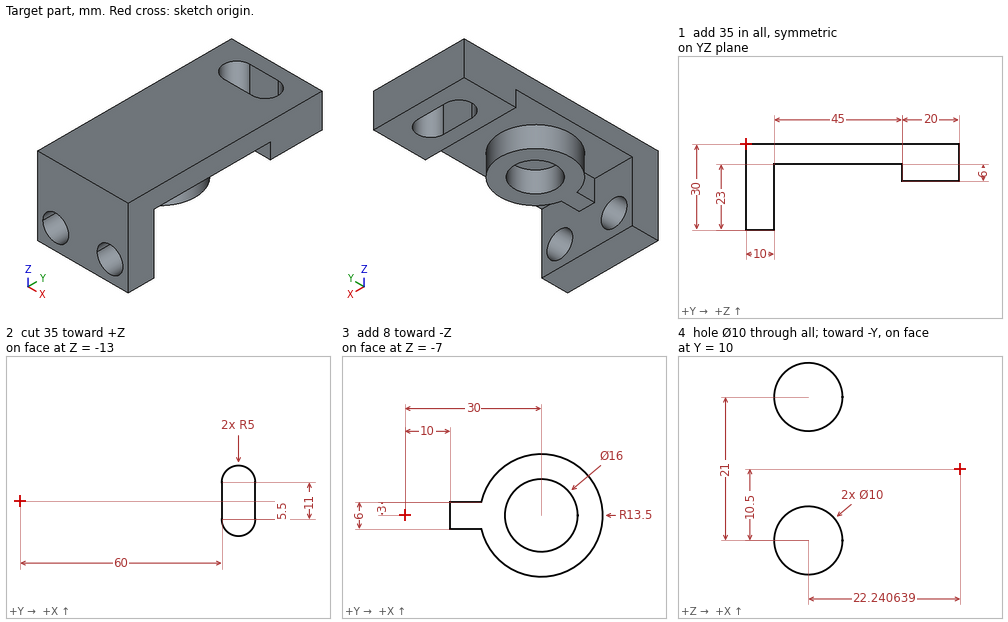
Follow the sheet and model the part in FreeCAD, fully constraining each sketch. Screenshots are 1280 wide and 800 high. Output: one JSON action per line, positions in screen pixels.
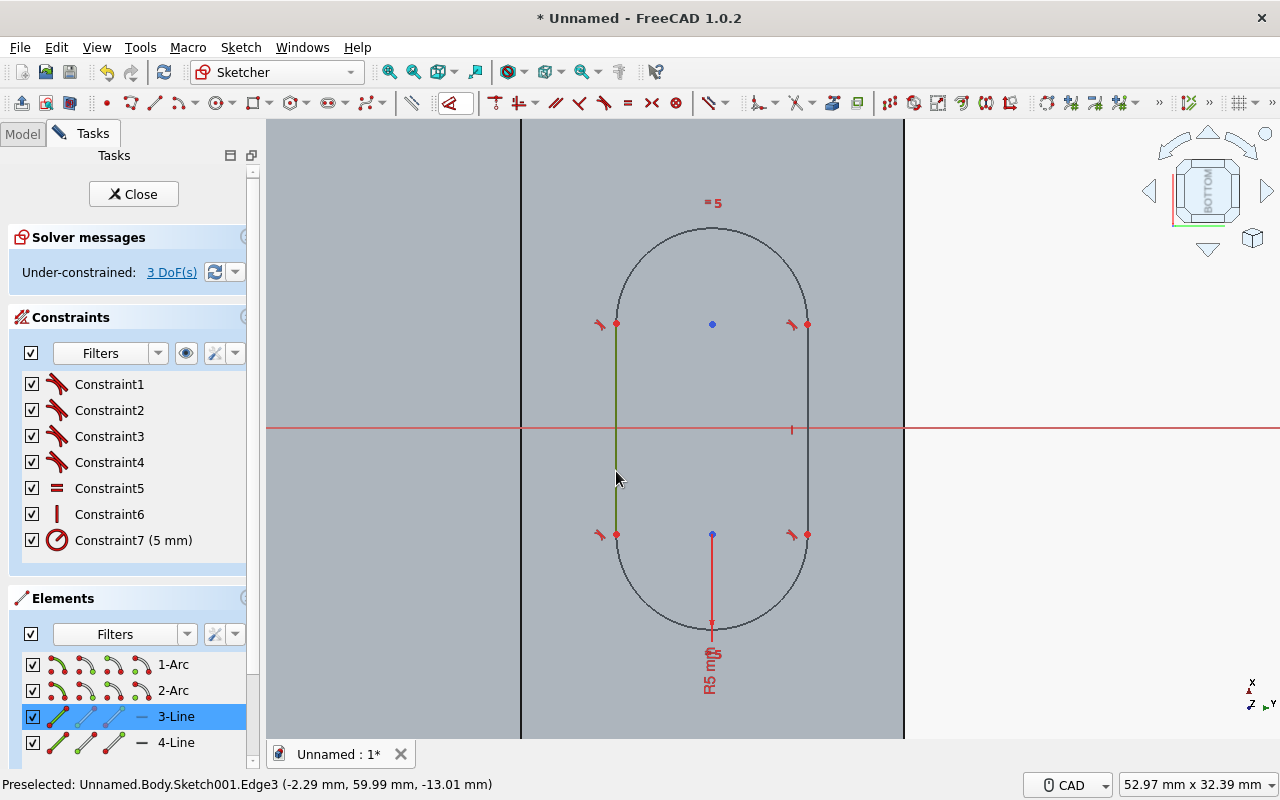
{"action": "left_click", "coordinate": [468, 104]}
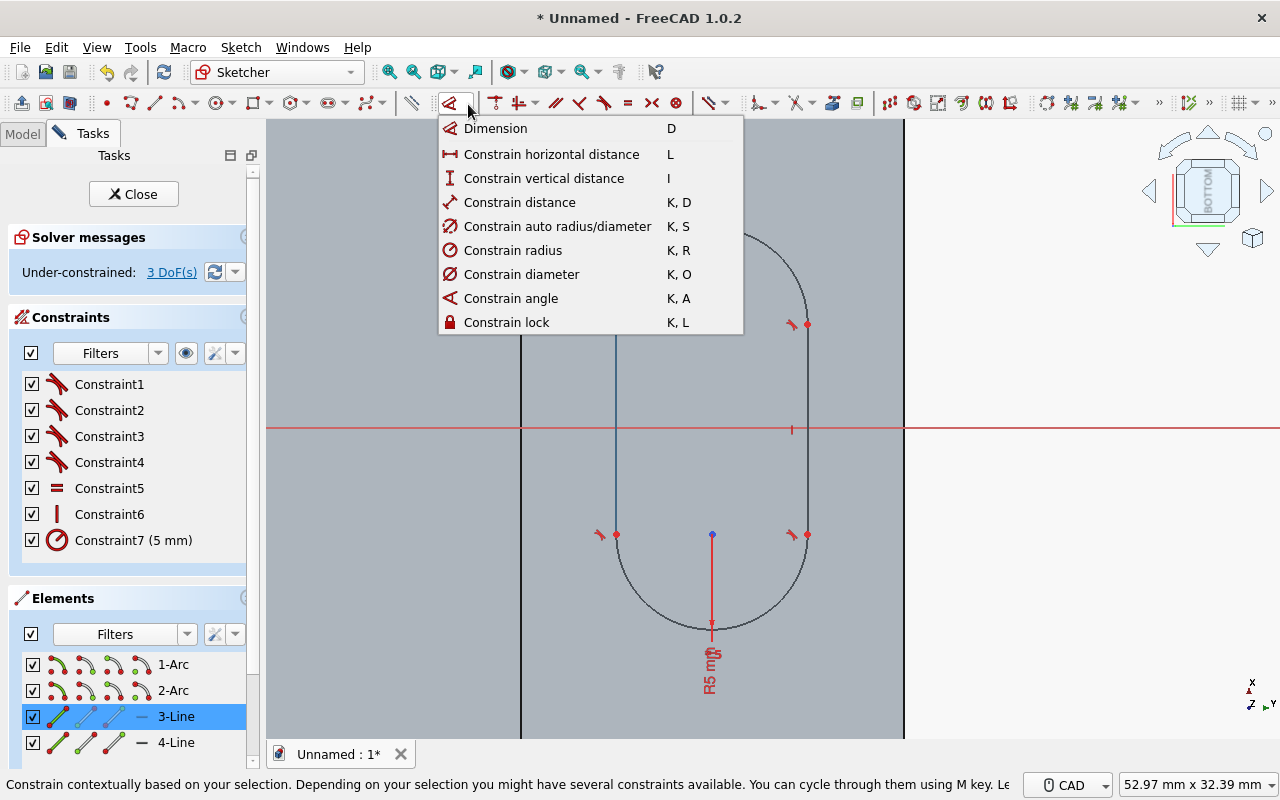
{"action": "left_click", "coordinate": [591, 178]}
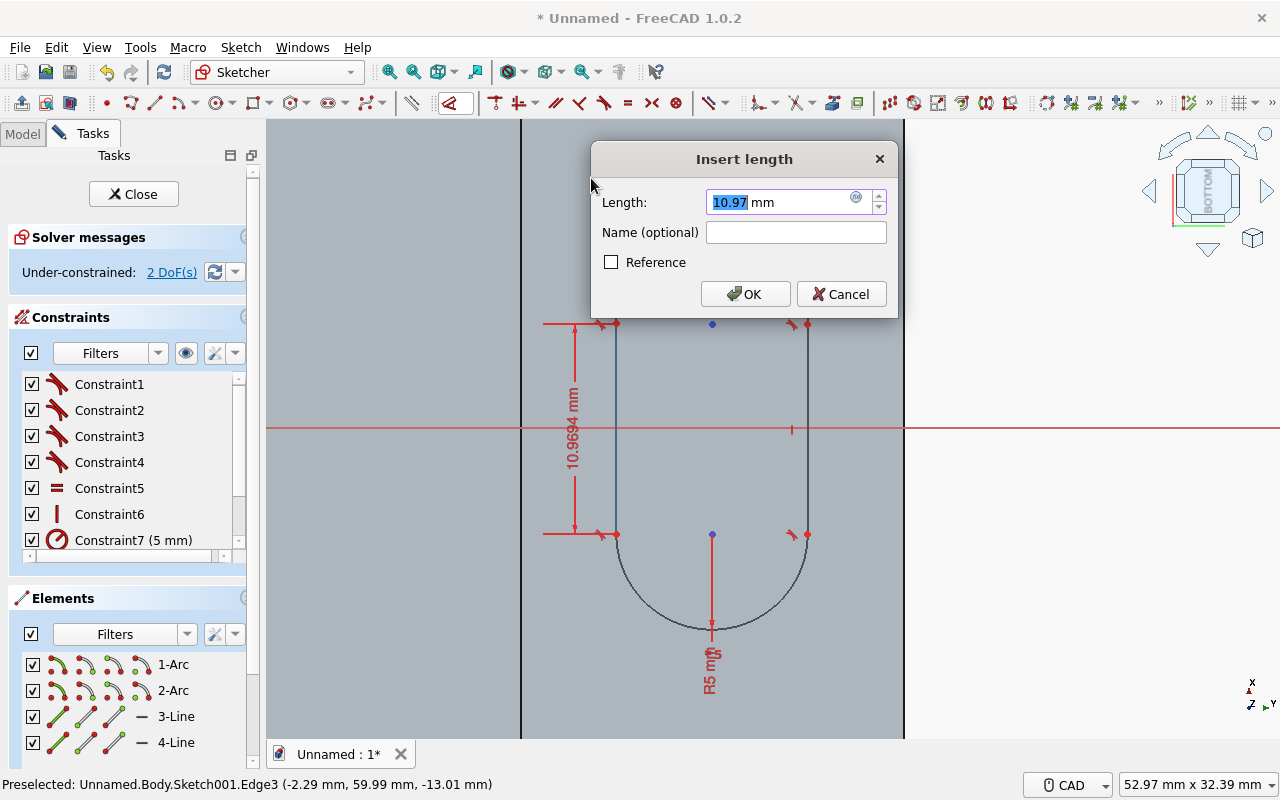
{"action": "type", "text": "11"}
{"action": "key", "text": "Return"}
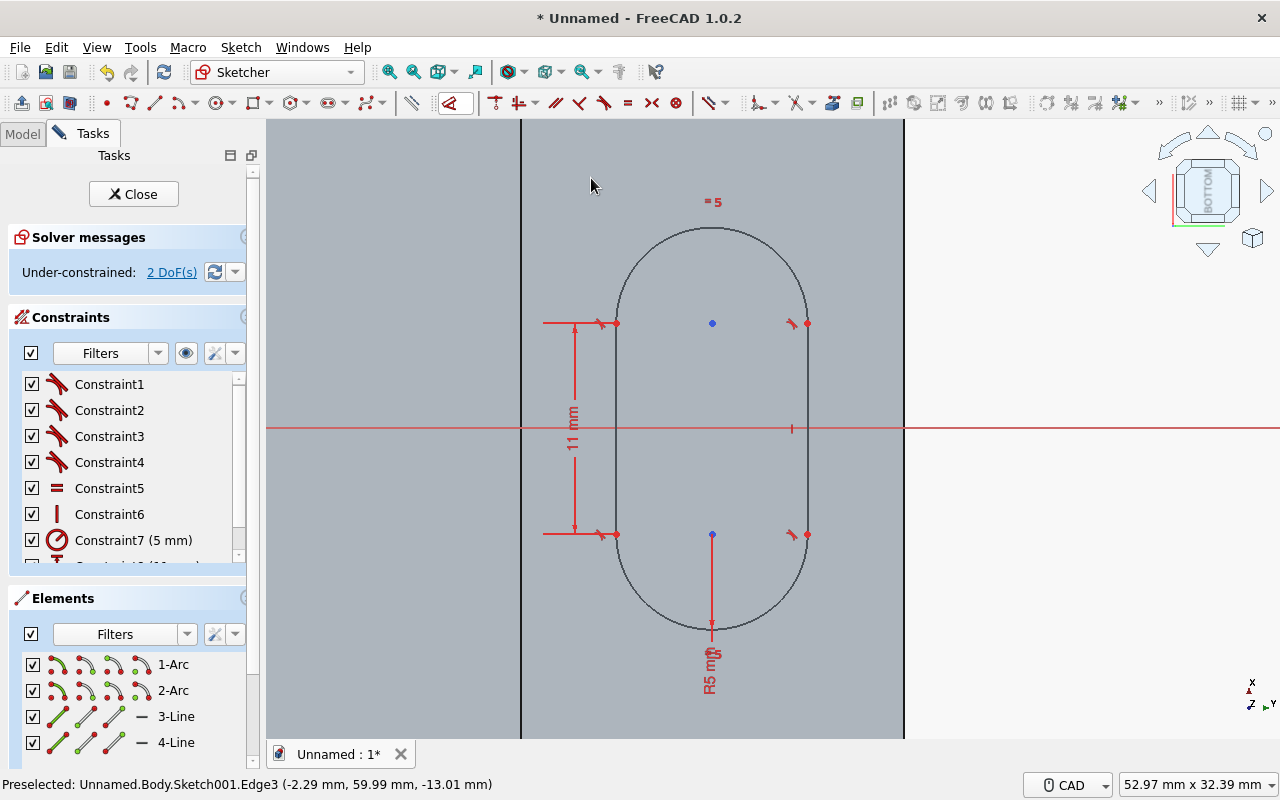
{"action": "left_click", "coordinate": [616, 534]}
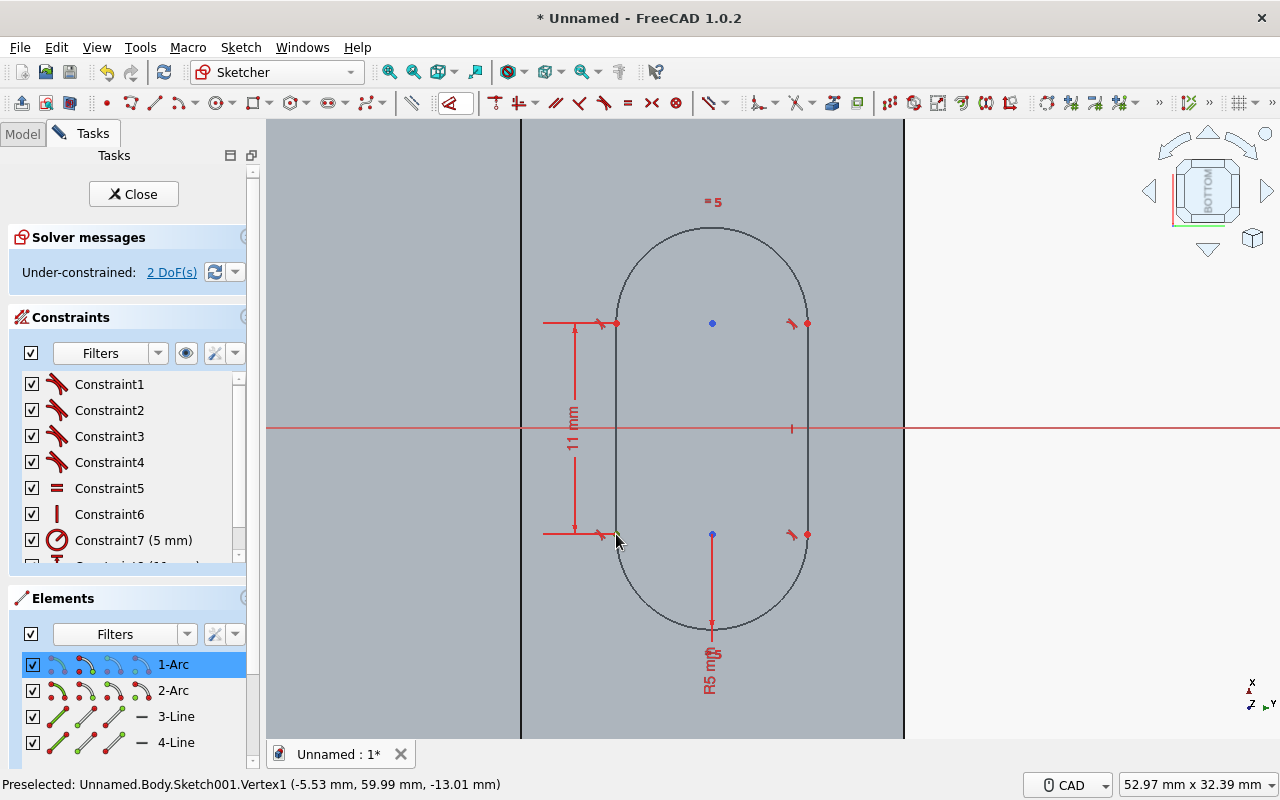
{"action": "left_click", "coordinate": [468, 104]}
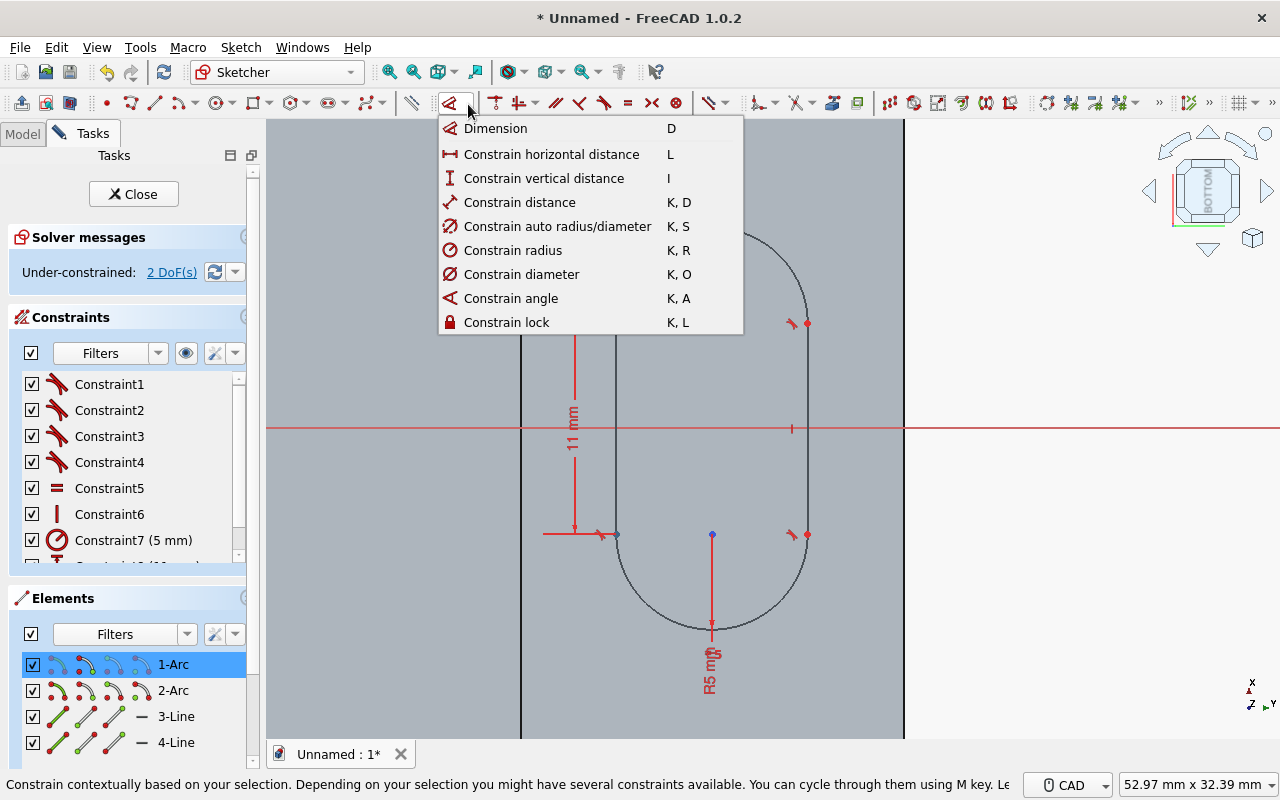
{"action": "left_click", "coordinate": [591, 154]}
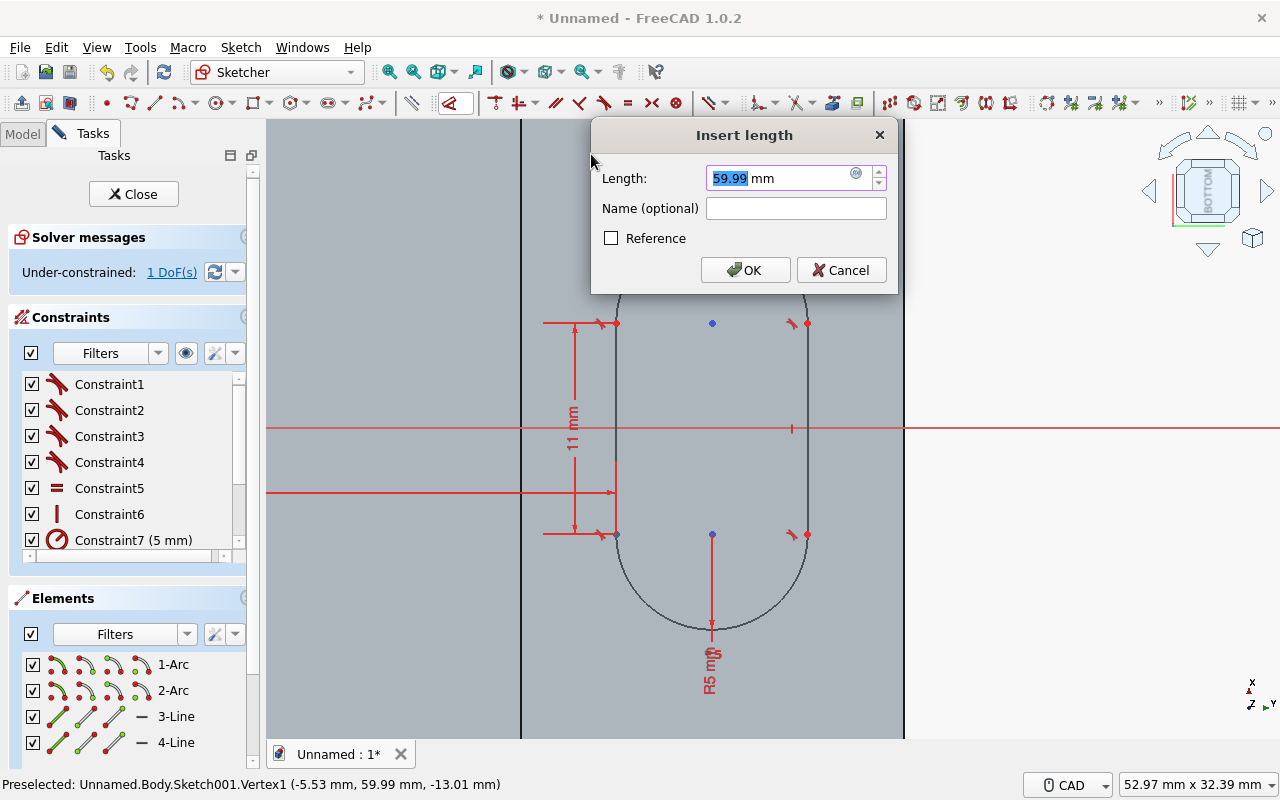
{"action": "type", "text": "60"}
{"action": "key", "text": "Return"}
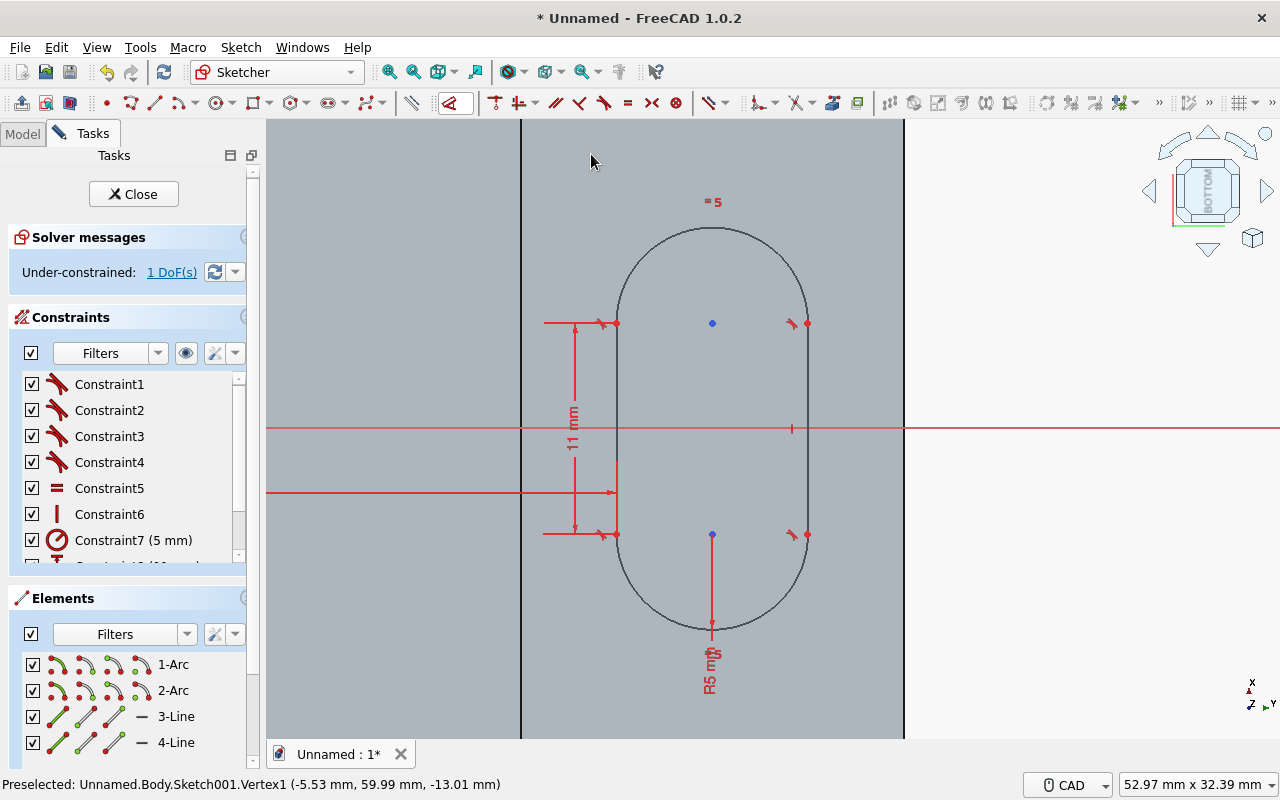
{"action": "left_click", "coordinate": [617, 534]}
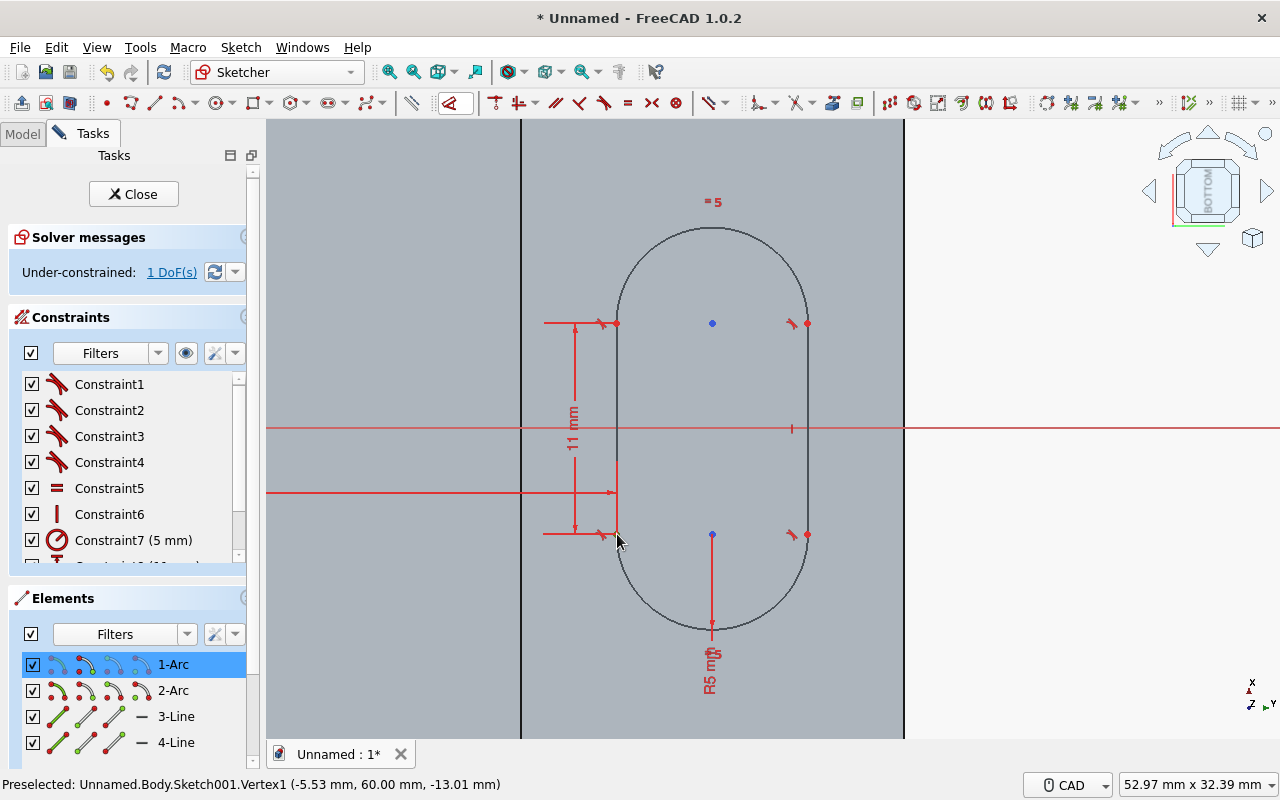
{"action": "key", "text": "i"}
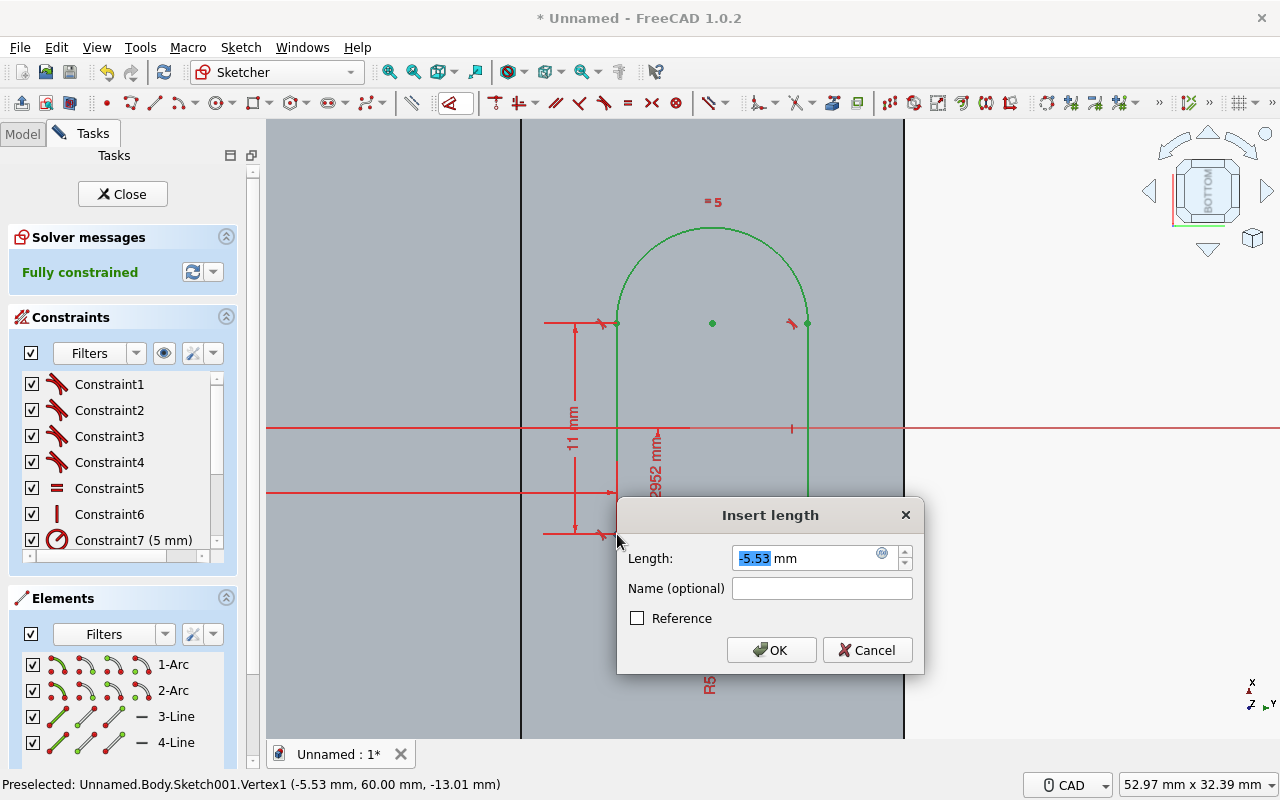
{"action": "type", "text": "-5.5"}
{"action": "key", "text": "Return"}